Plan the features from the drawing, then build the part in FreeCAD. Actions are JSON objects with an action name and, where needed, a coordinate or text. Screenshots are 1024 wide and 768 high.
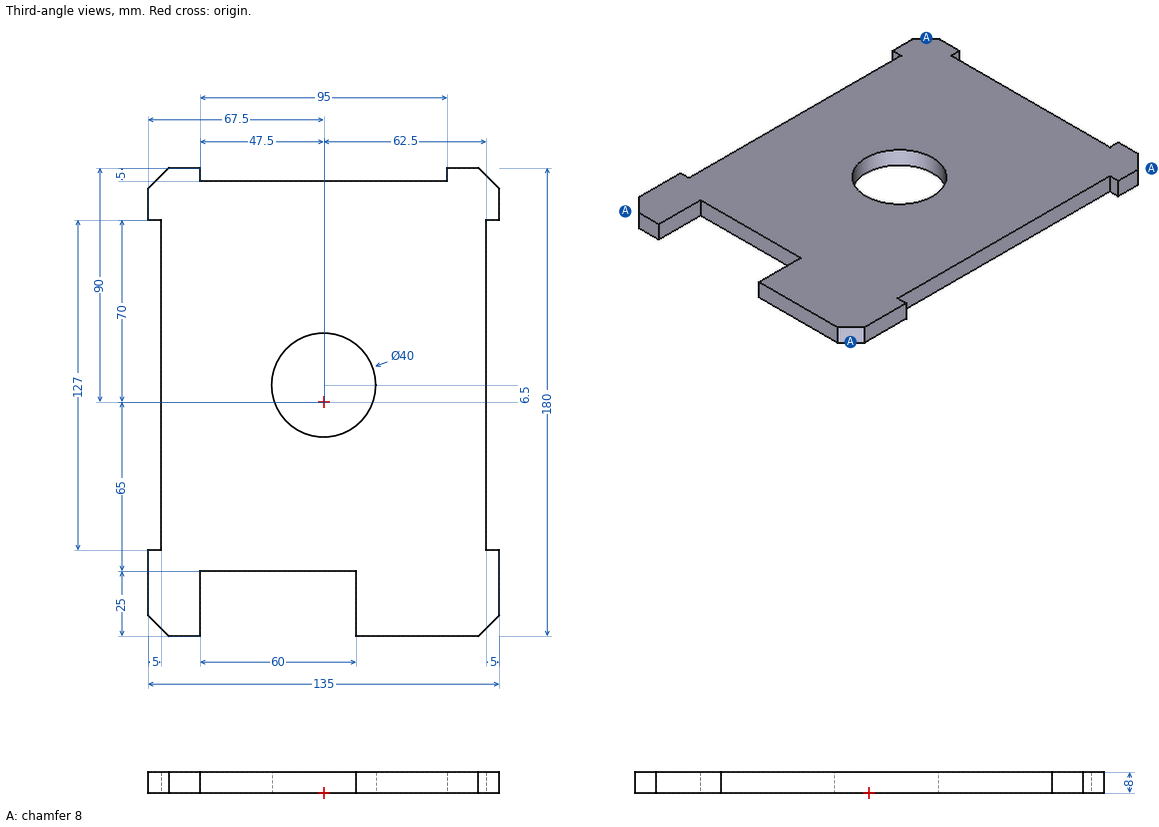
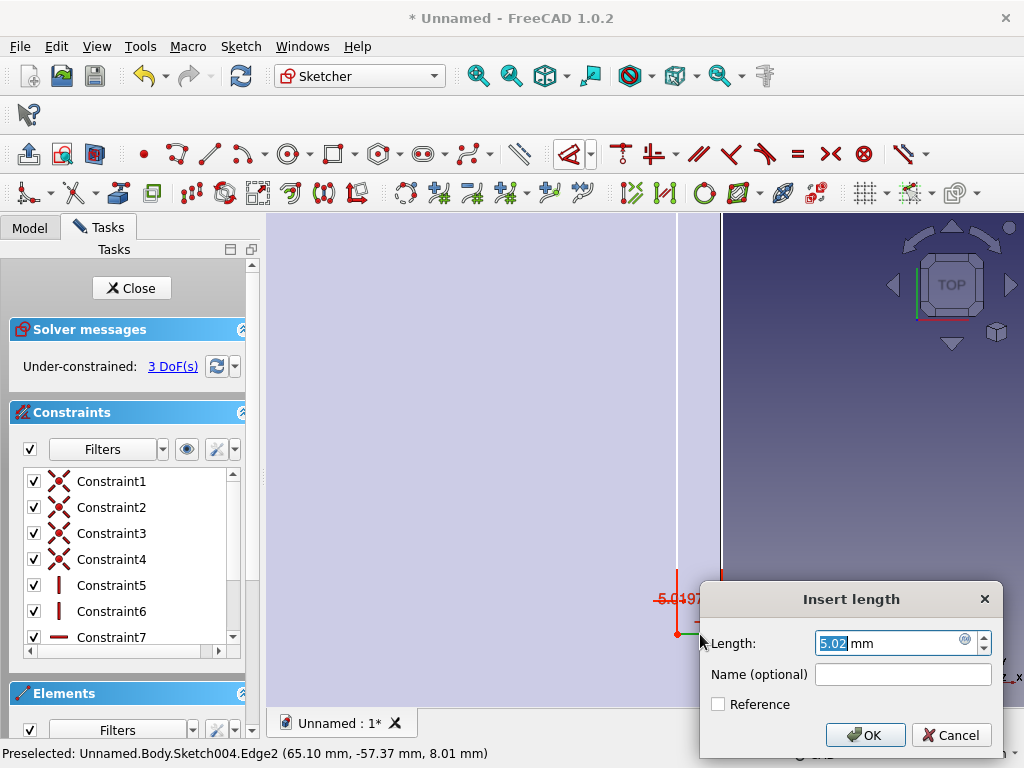
{"action": "type", "text": "5"}
{"action": "key", "text": "Return"}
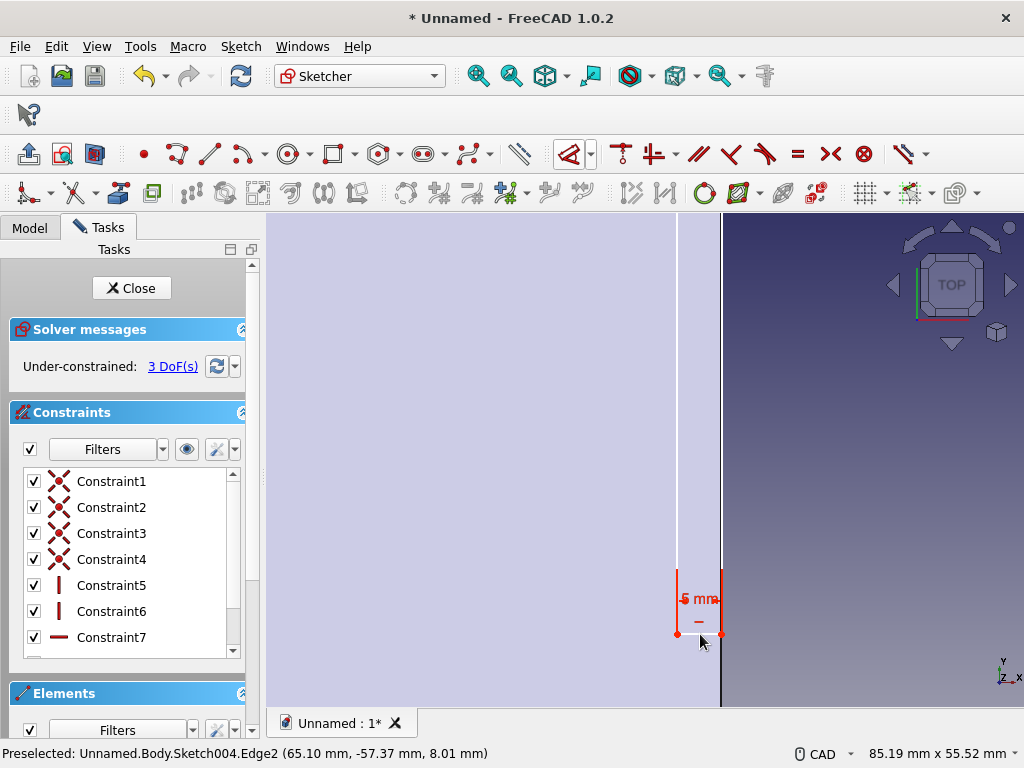
{"action": "scroll", "coordinate": [643, 630], "scroll_direction": "down", "scroll_amount": 6}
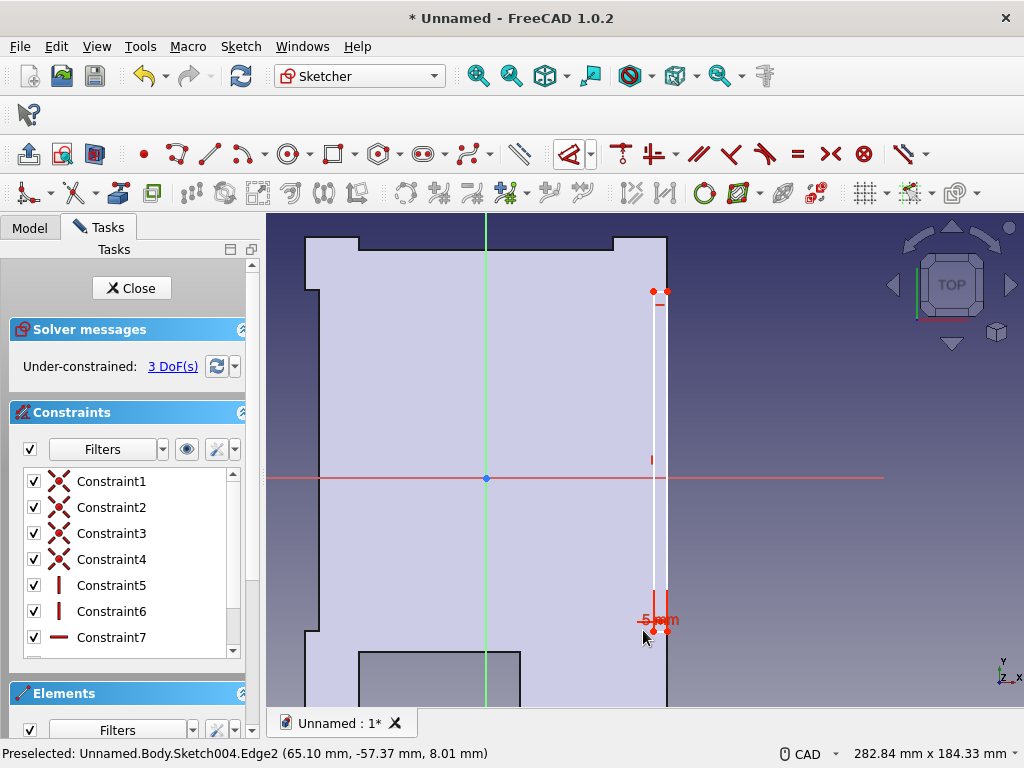
{"action": "left_click", "coordinate": [654, 530]}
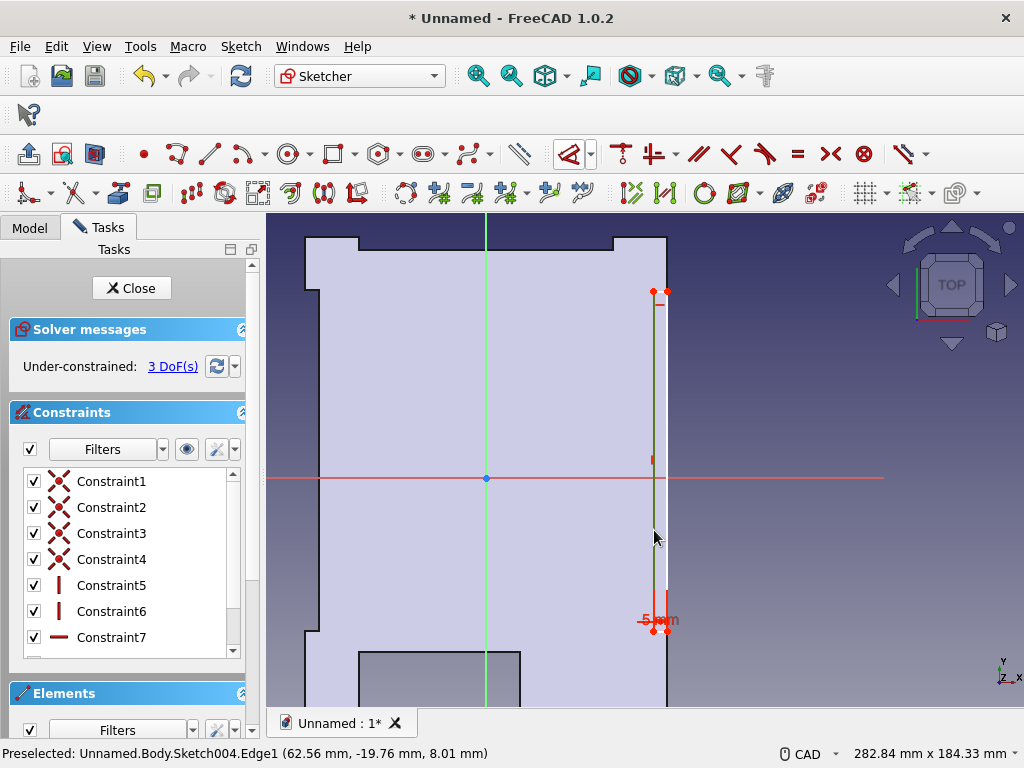
{"action": "key", "text": "i"}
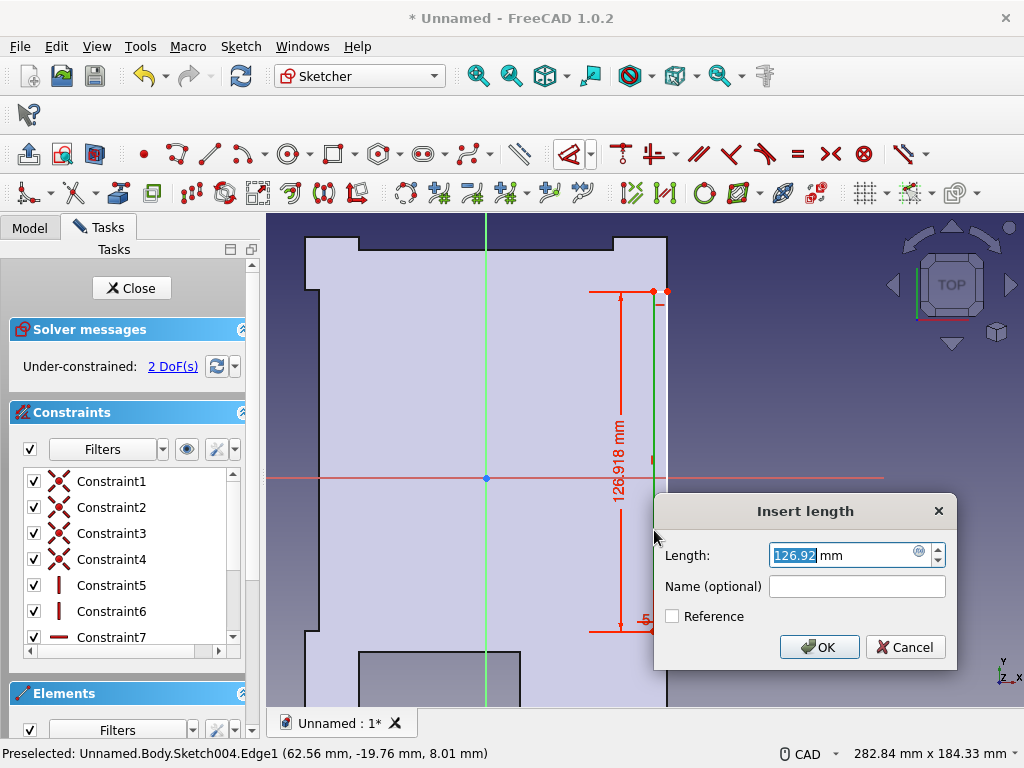
{"action": "type", "text": "127"}
{"action": "key", "text": "Return"}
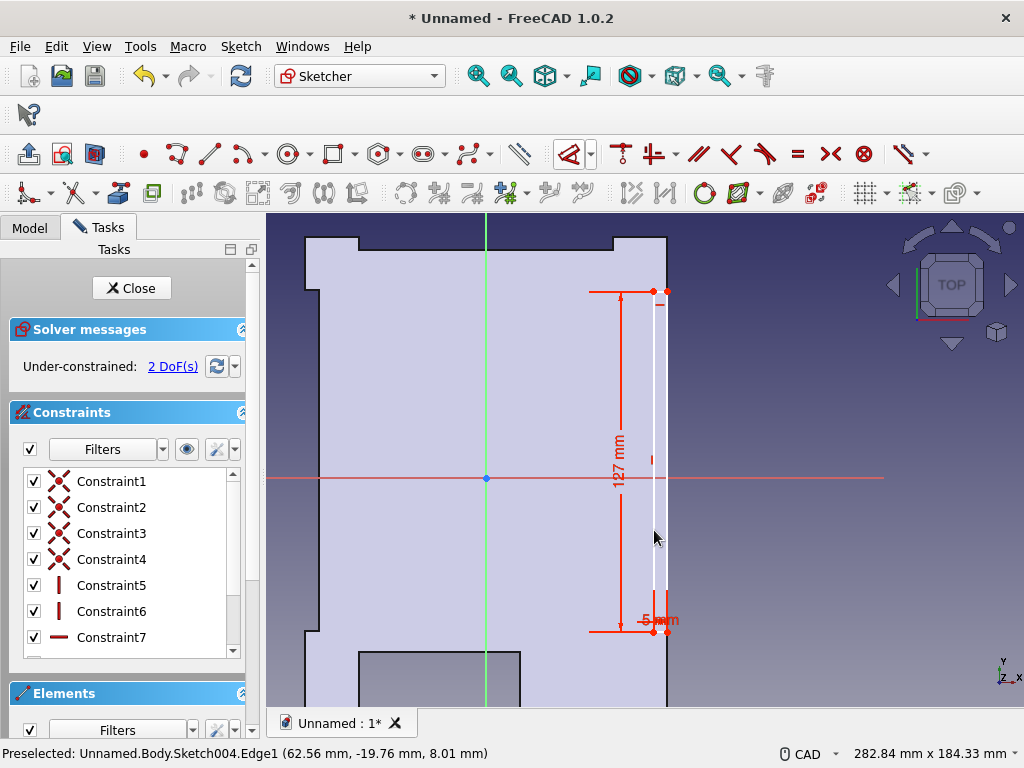
{"action": "left_click", "coordinate": [654, 292]}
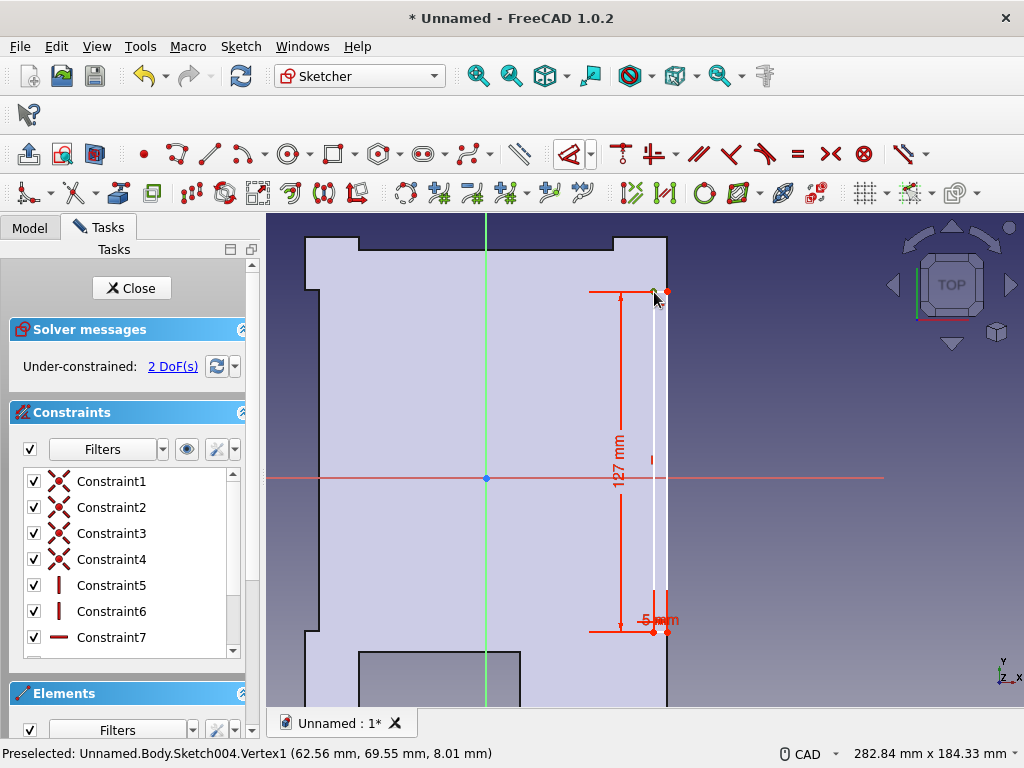
{"action": "key", "text": "i"}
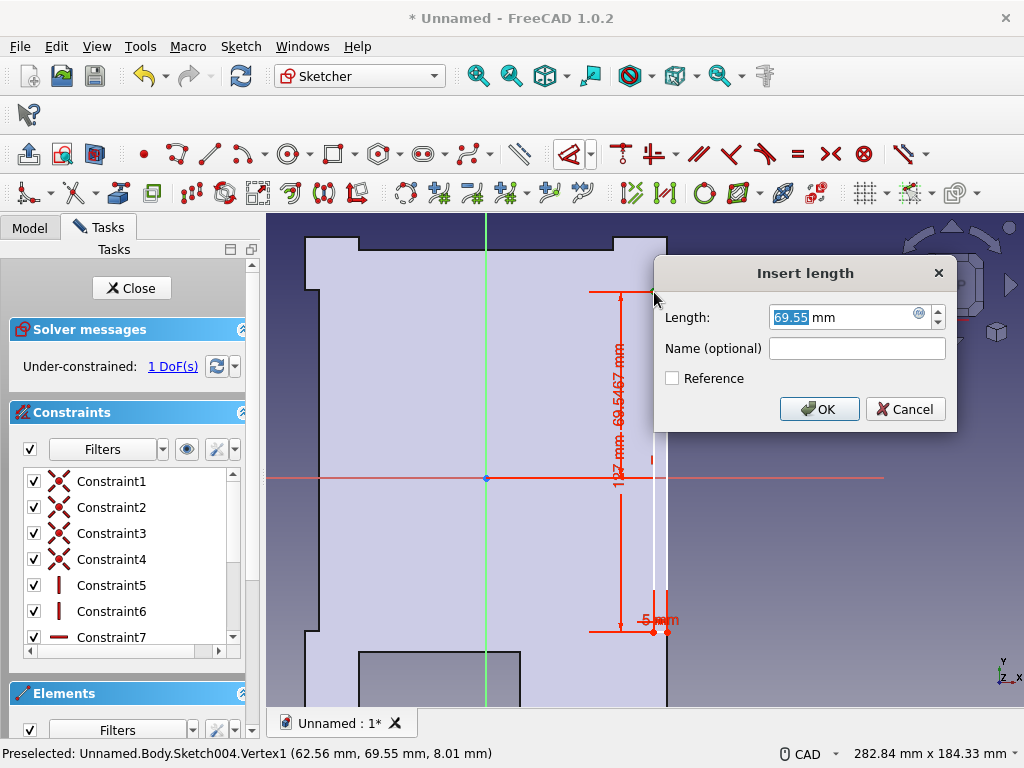
{"action": "type", "text": "70"}
{"action": "key", "text": "Return"}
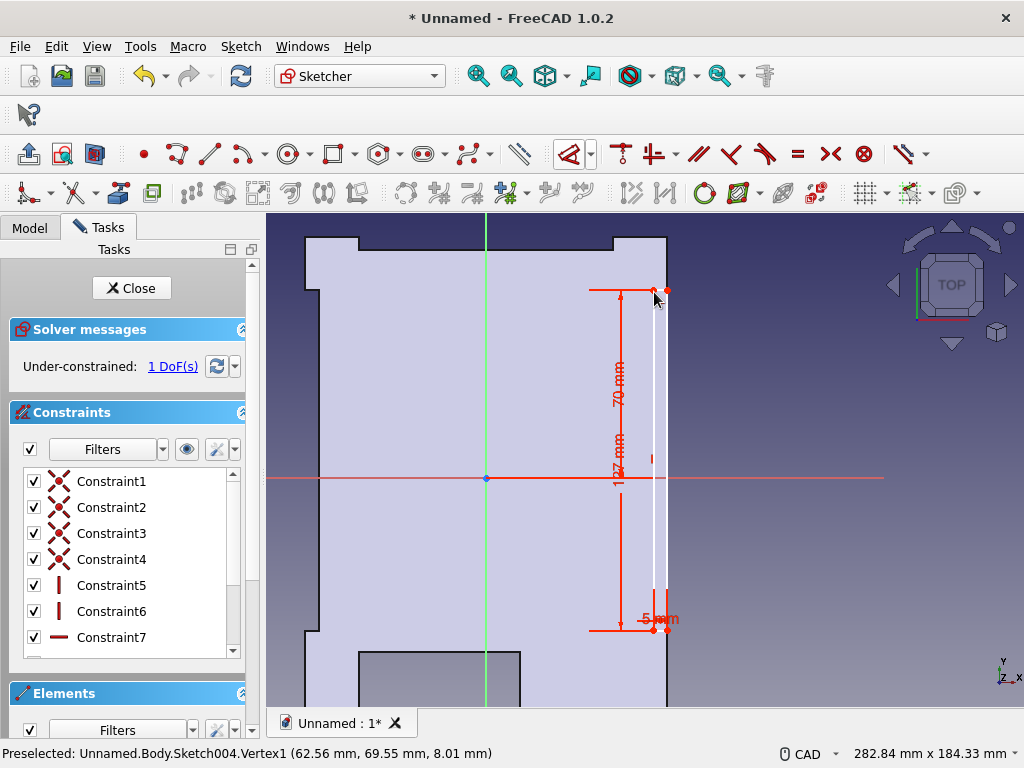
{"action": "left_click", "coordinate": [654, 290]}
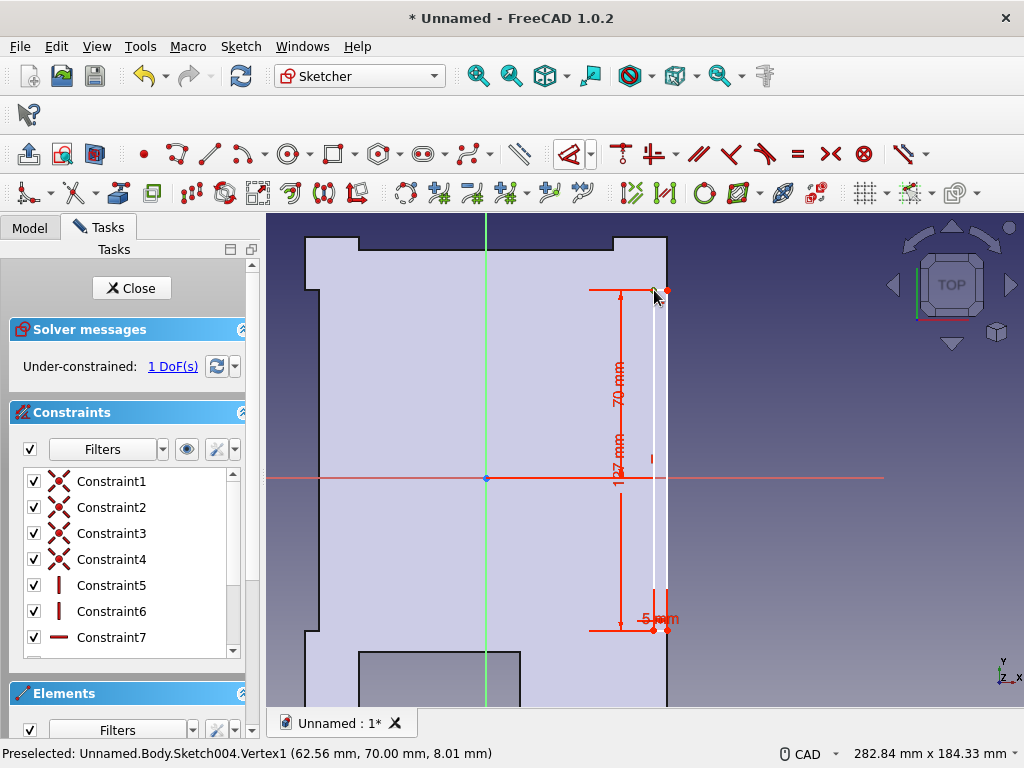
{"action": "key", "text": "l"}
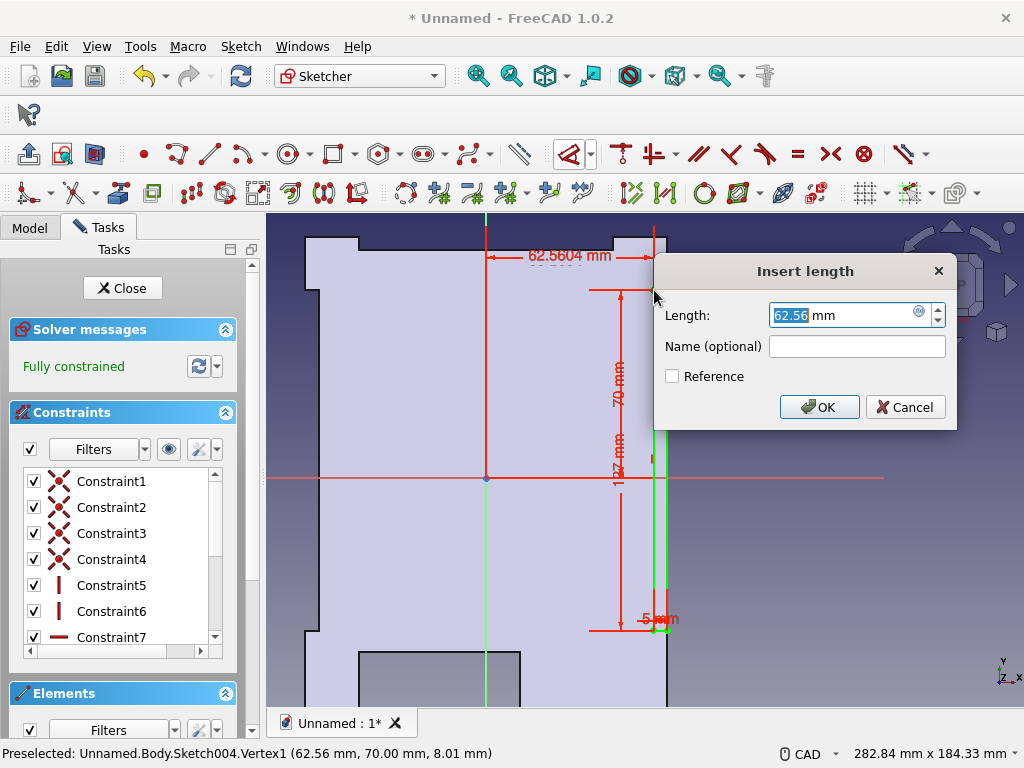
{"action": "type", "text": "62.5"}
{"action": "key", "text": "Return"}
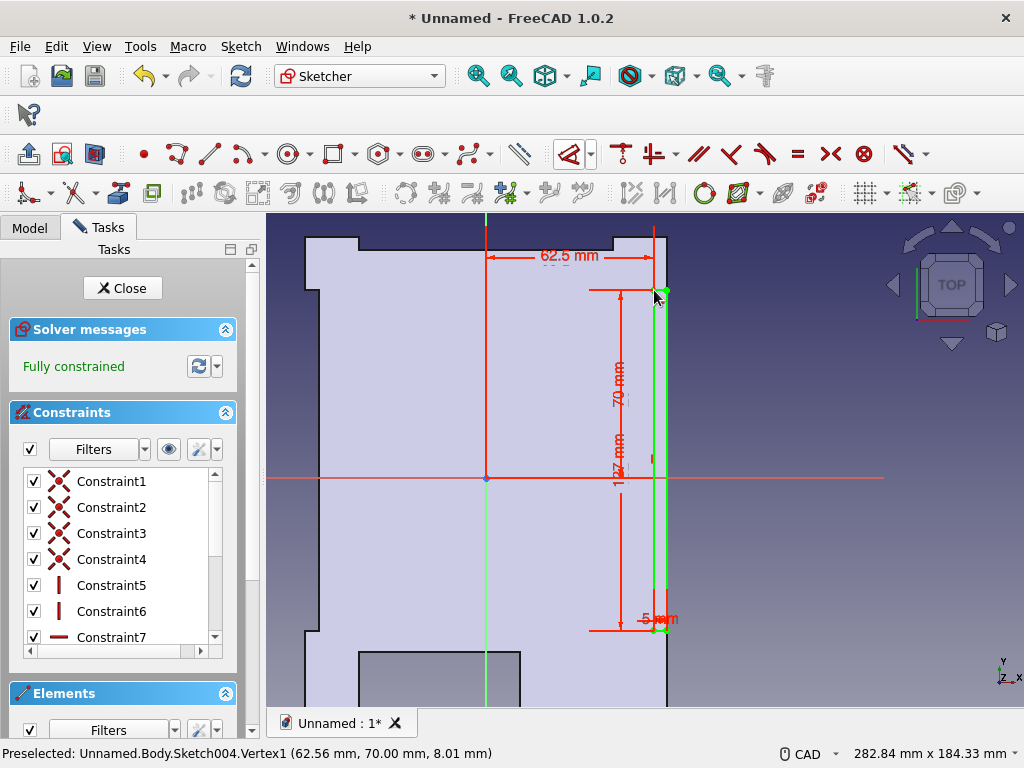
{"action": "left_click", "coordinate": [123, 288]}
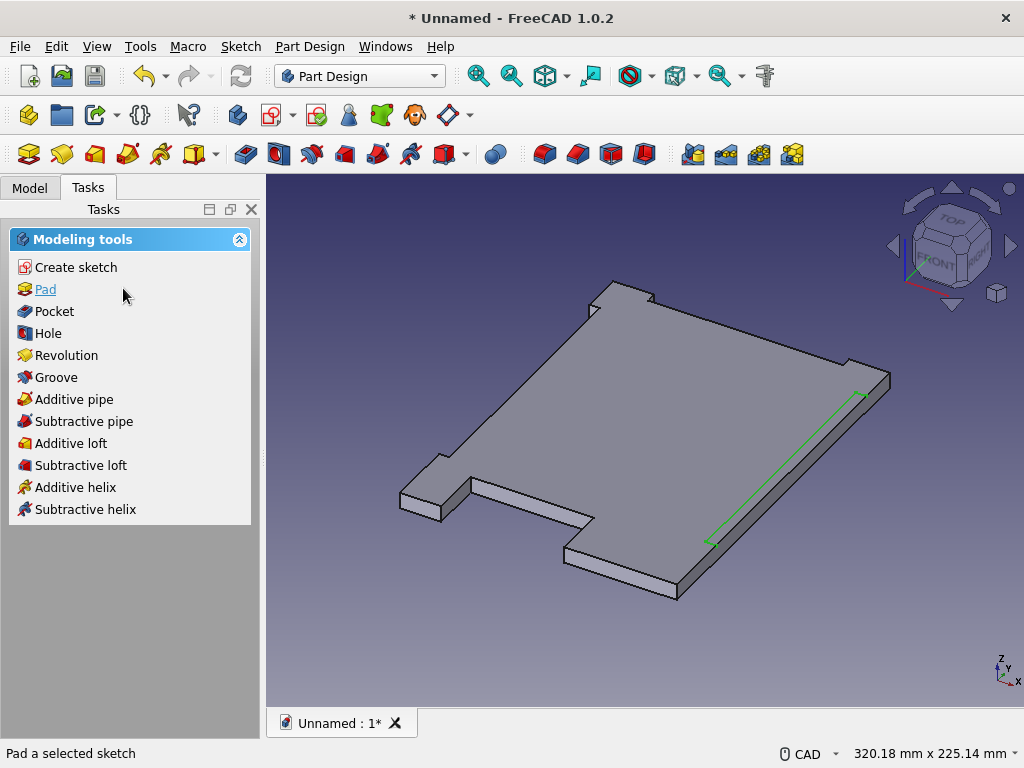
{"action": "left_click", "coordinate": [246, 154]}